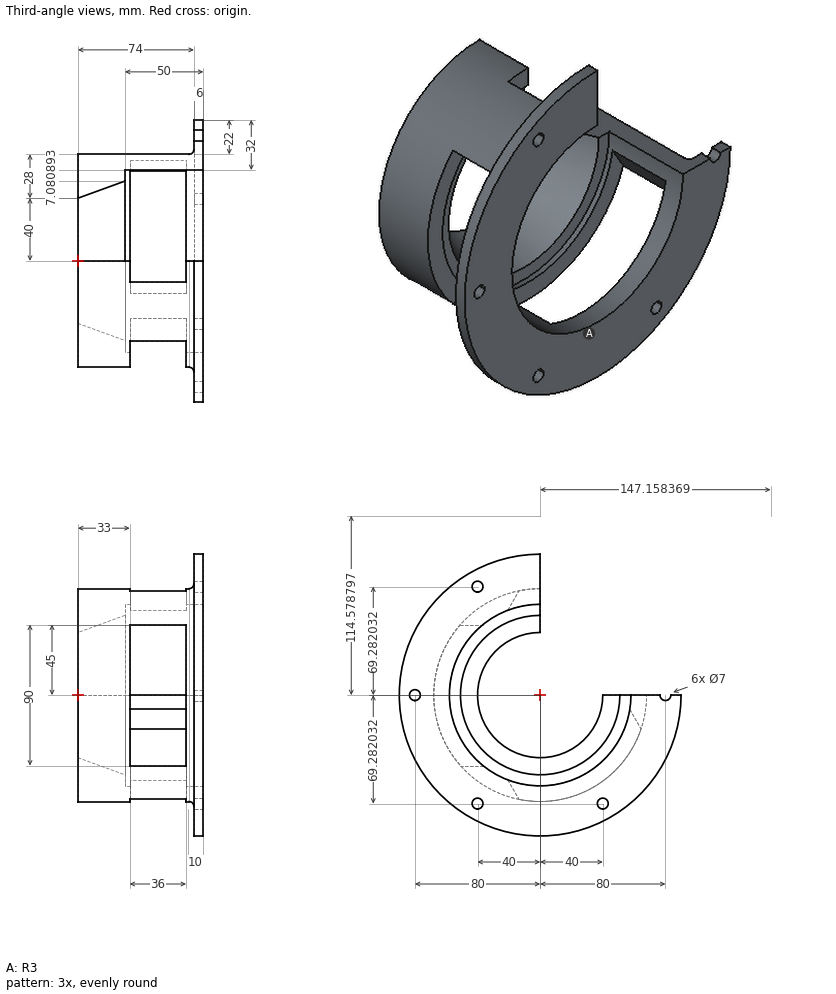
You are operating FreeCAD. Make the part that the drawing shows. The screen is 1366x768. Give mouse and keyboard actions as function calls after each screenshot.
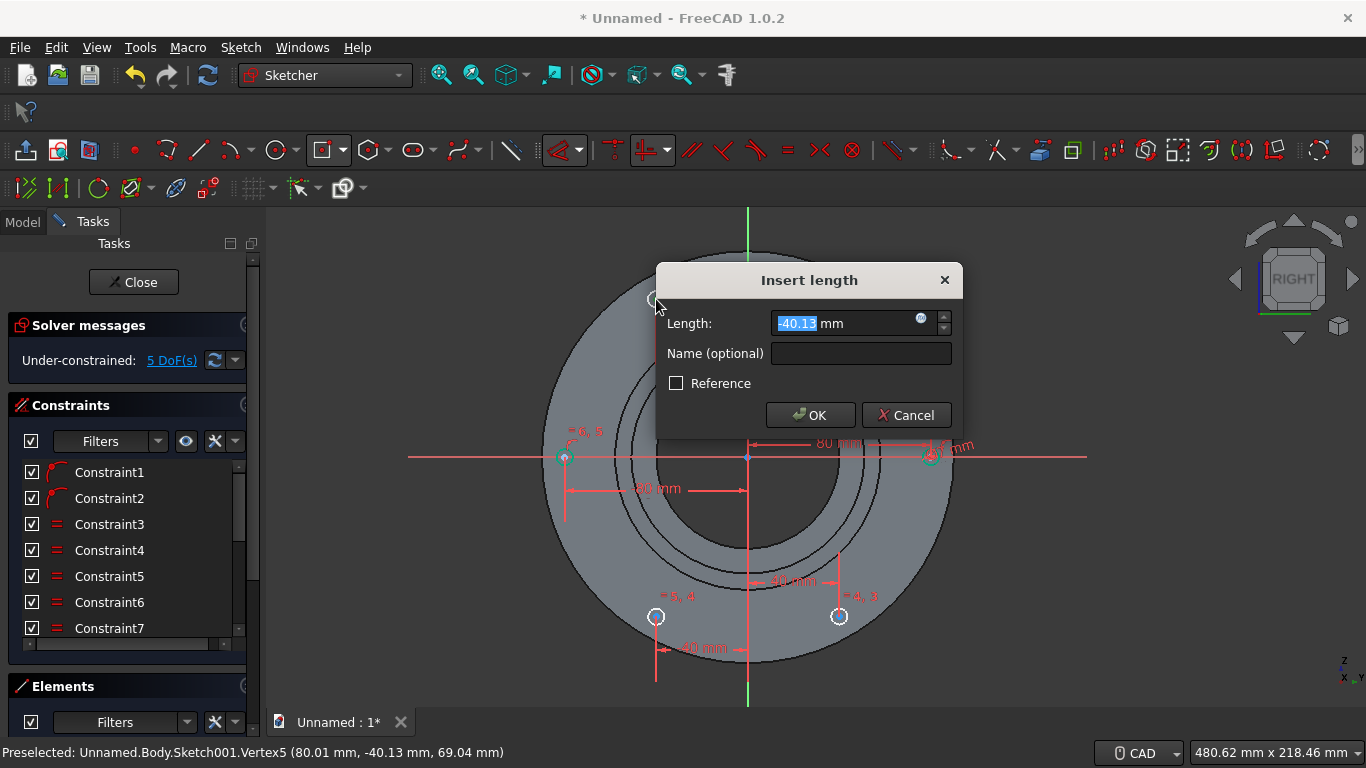
text(-40)
key(Return)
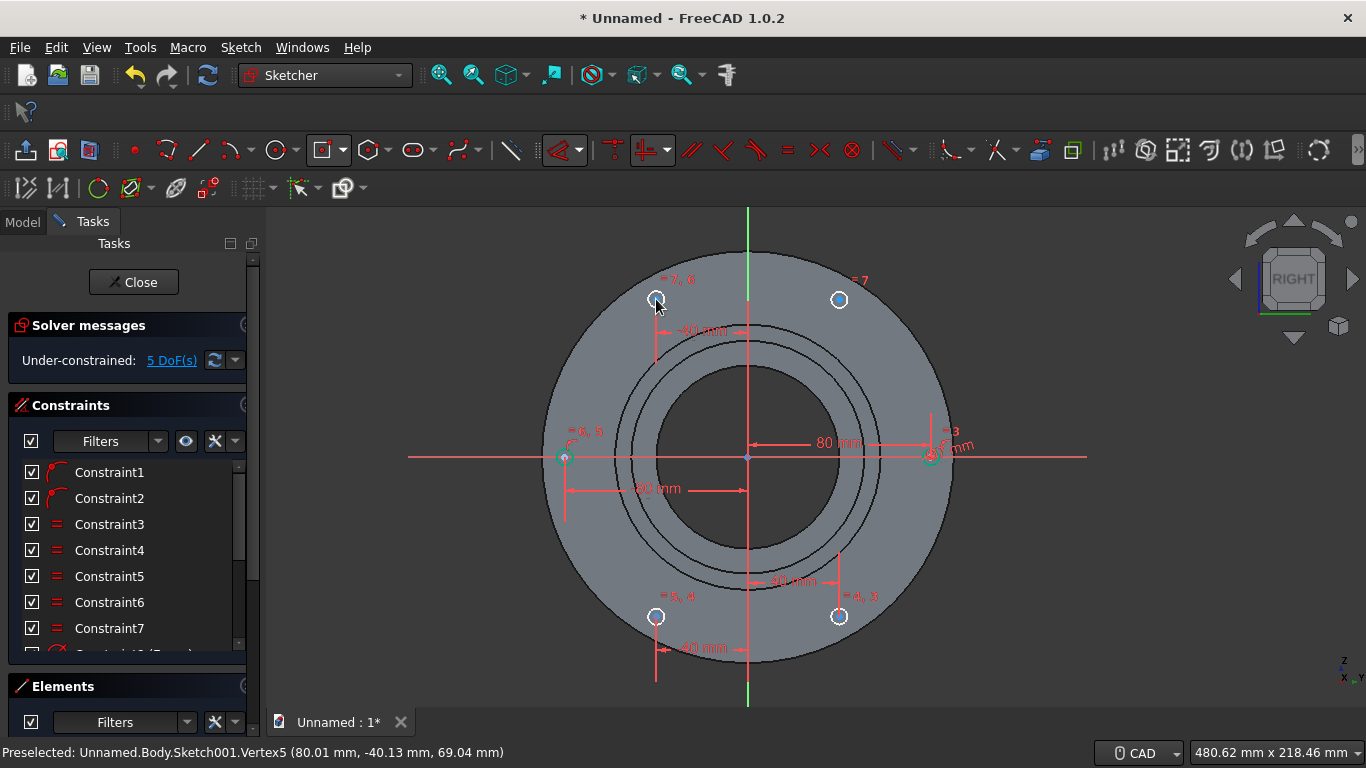
click(839, 300)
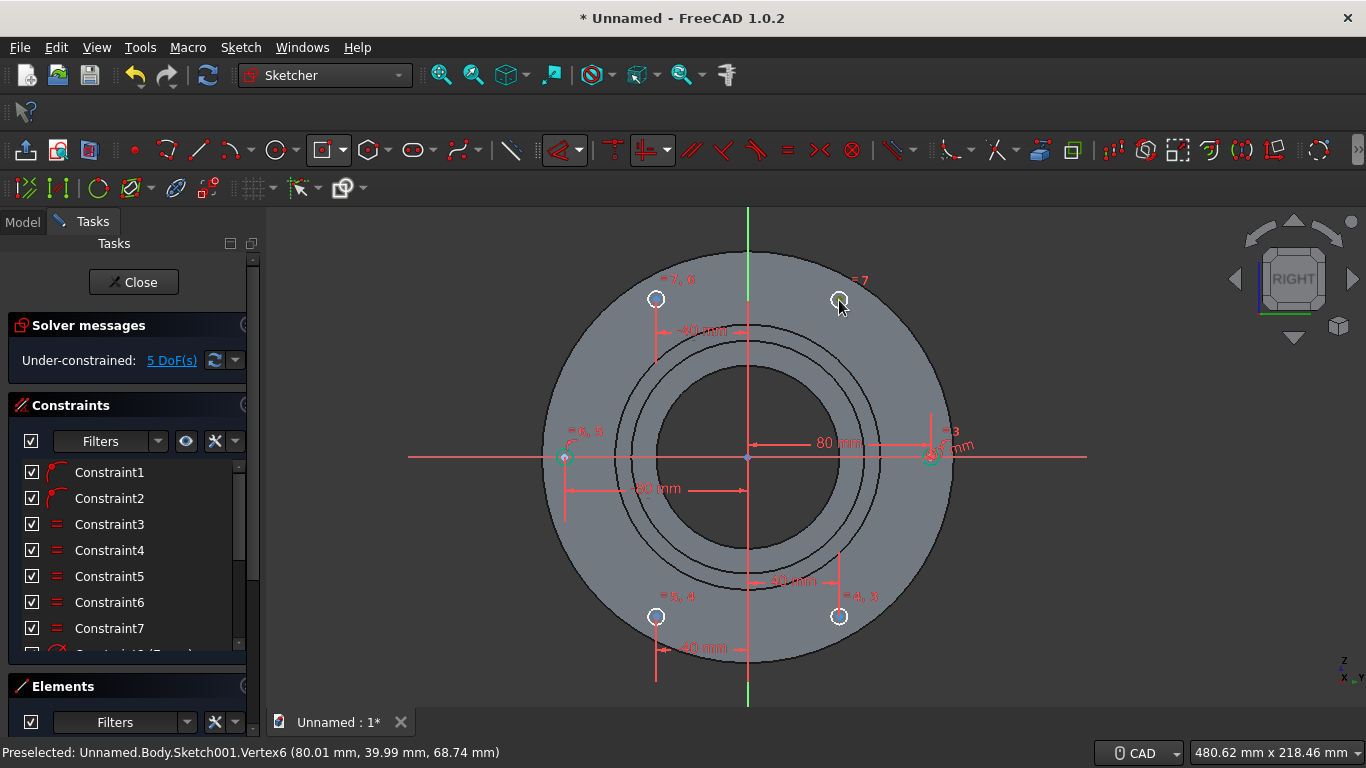
key(l)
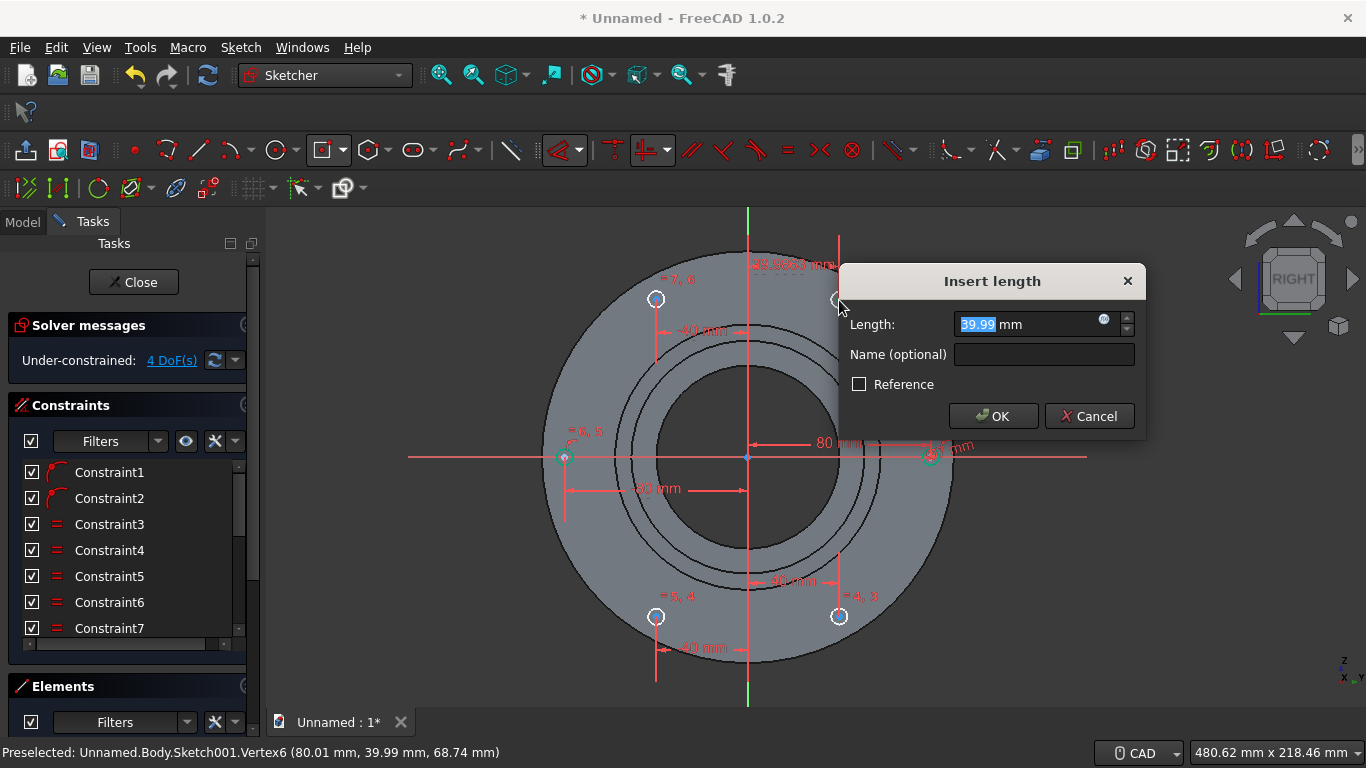
text(40)
key(Return)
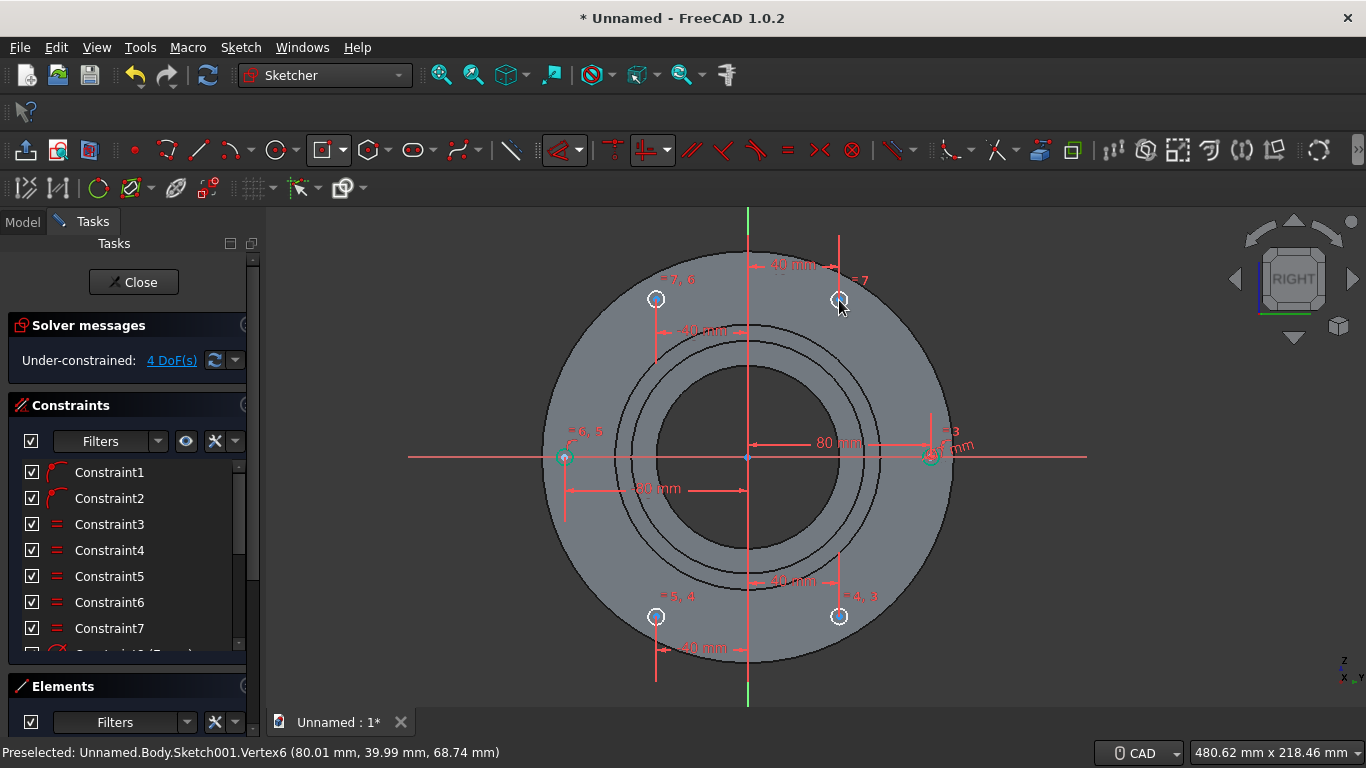
click(839, 616)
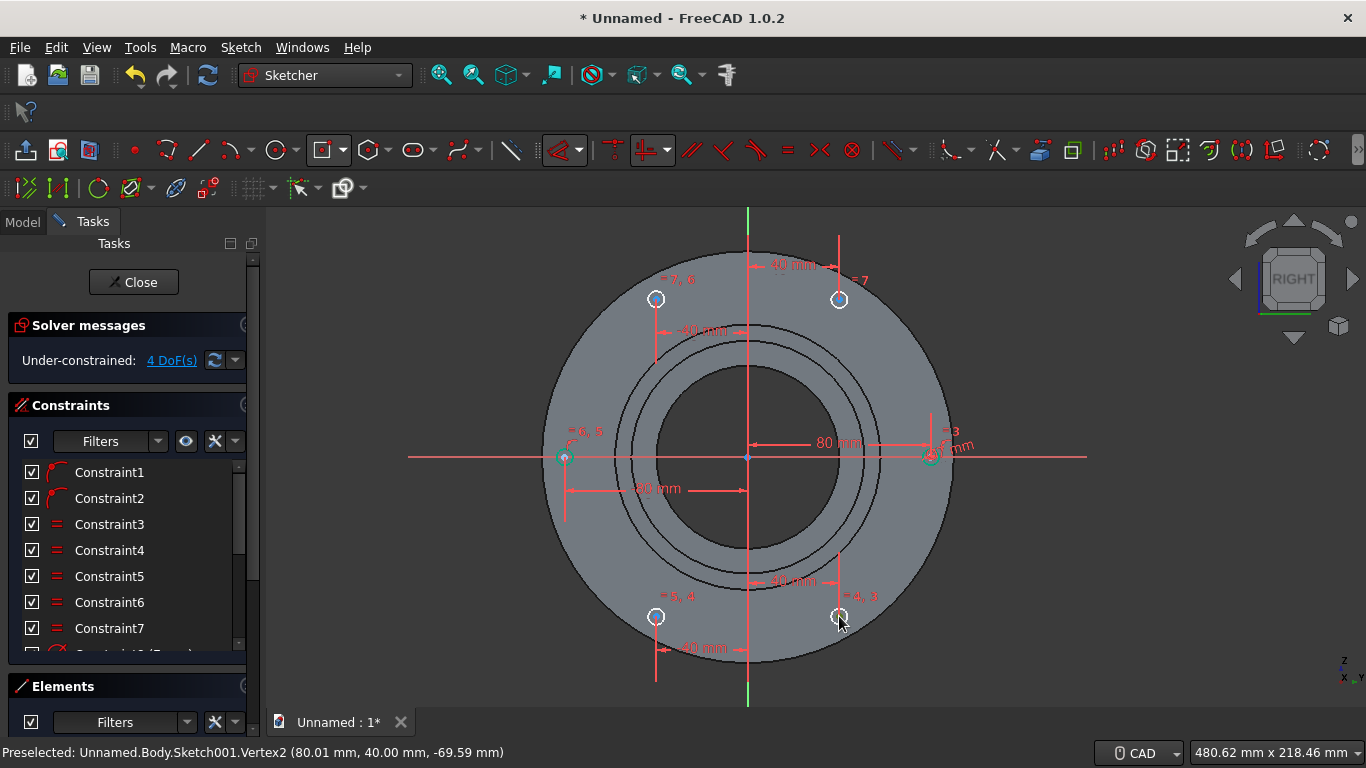
click(582, 150)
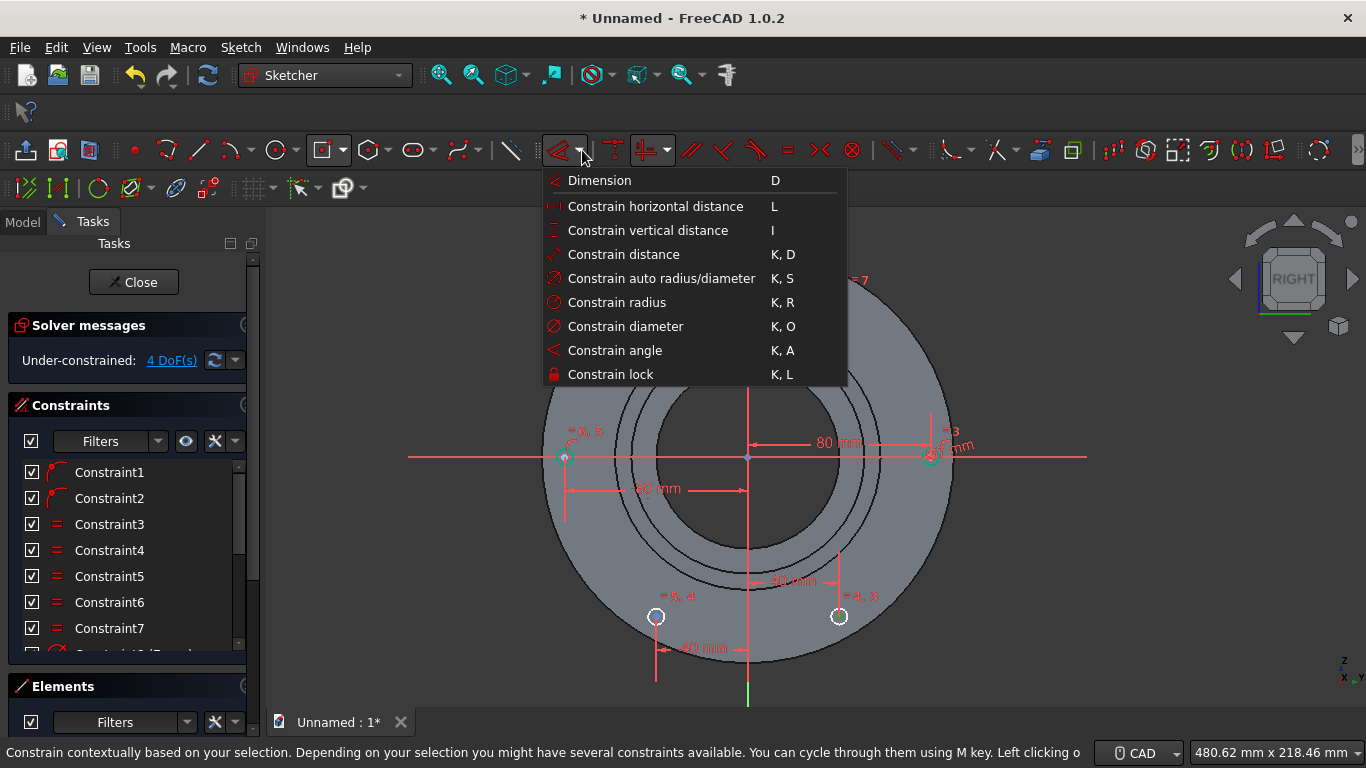
click(695, 230)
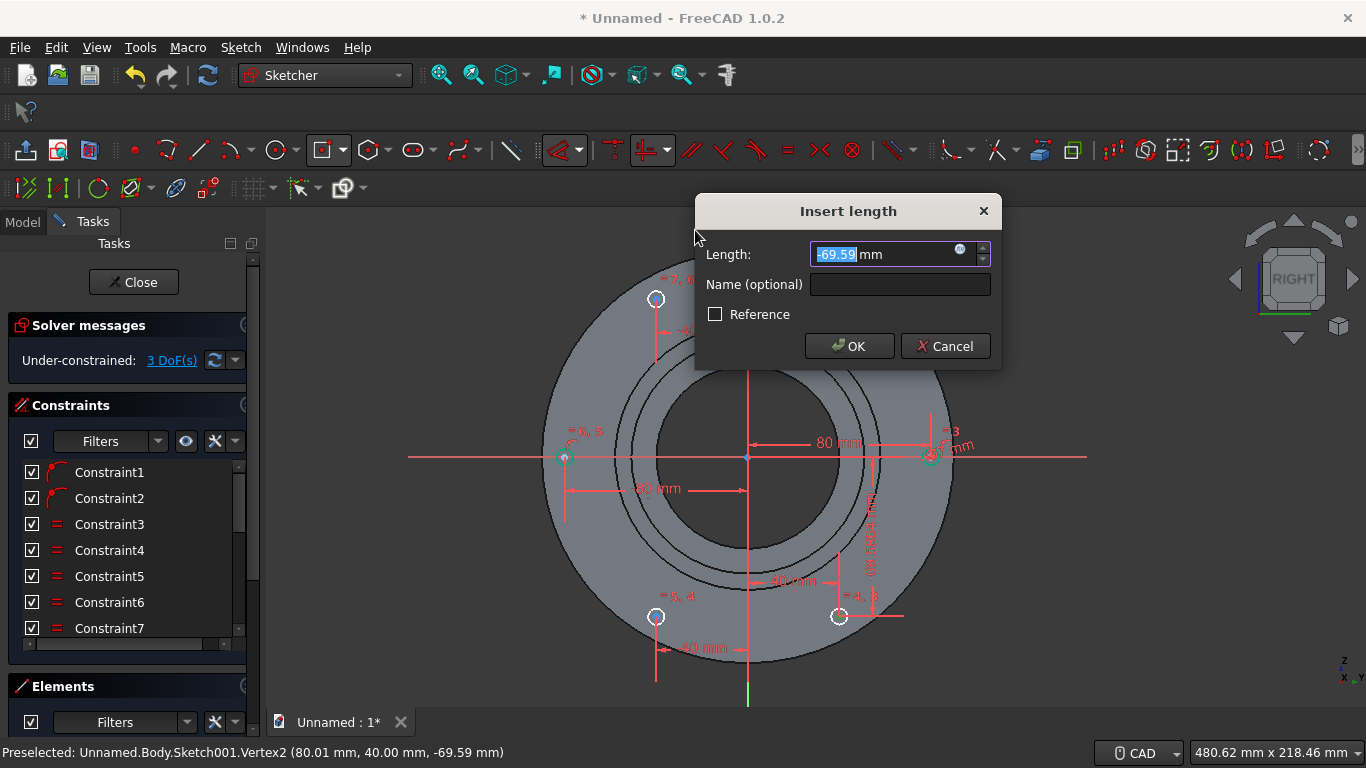
text(-69.282032)
key(Return)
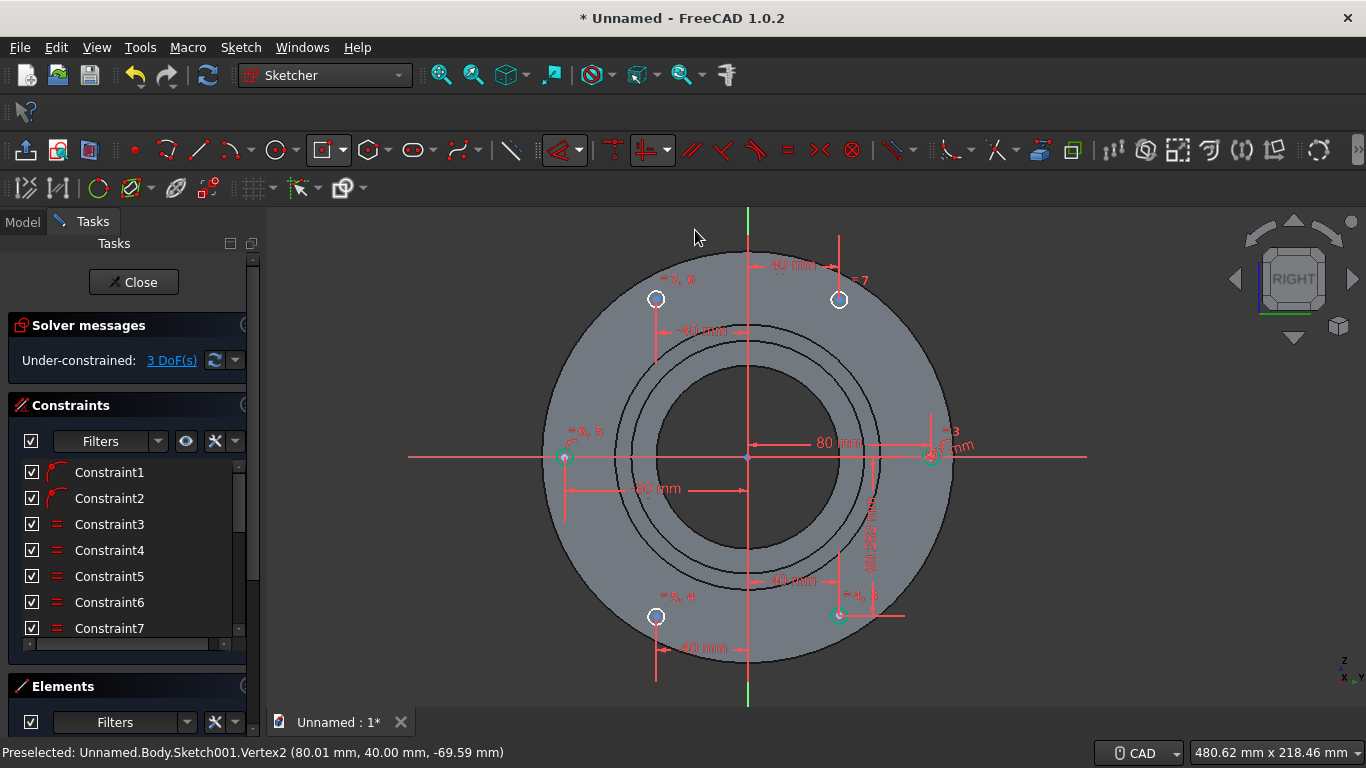
click(656, 617)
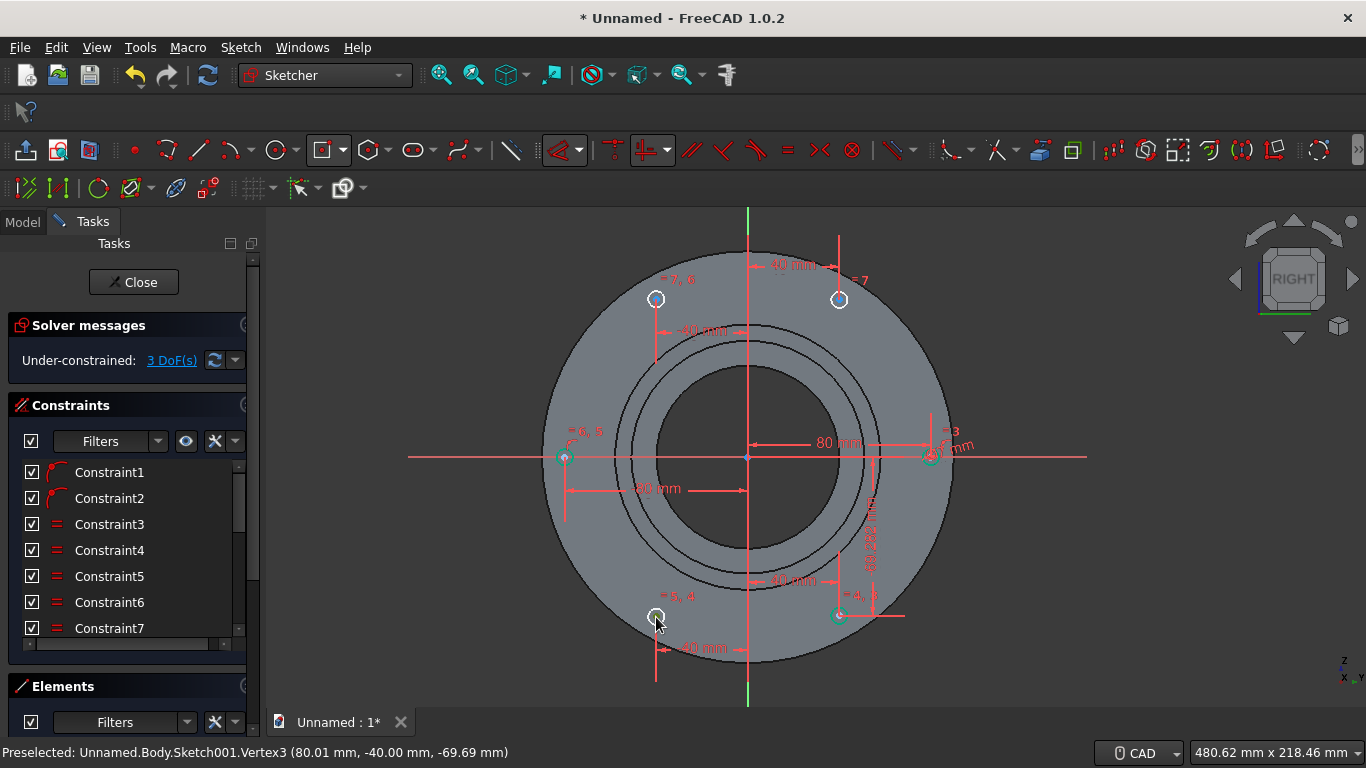
key(i)